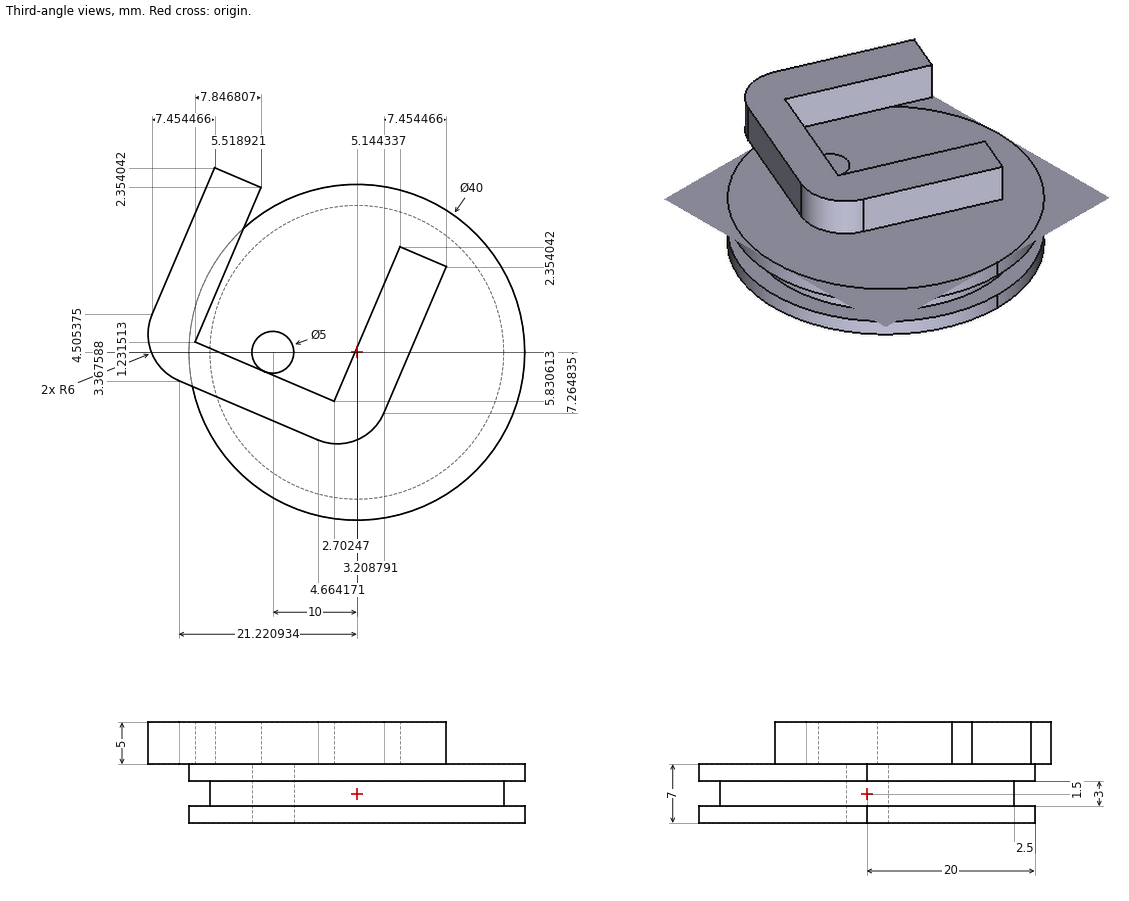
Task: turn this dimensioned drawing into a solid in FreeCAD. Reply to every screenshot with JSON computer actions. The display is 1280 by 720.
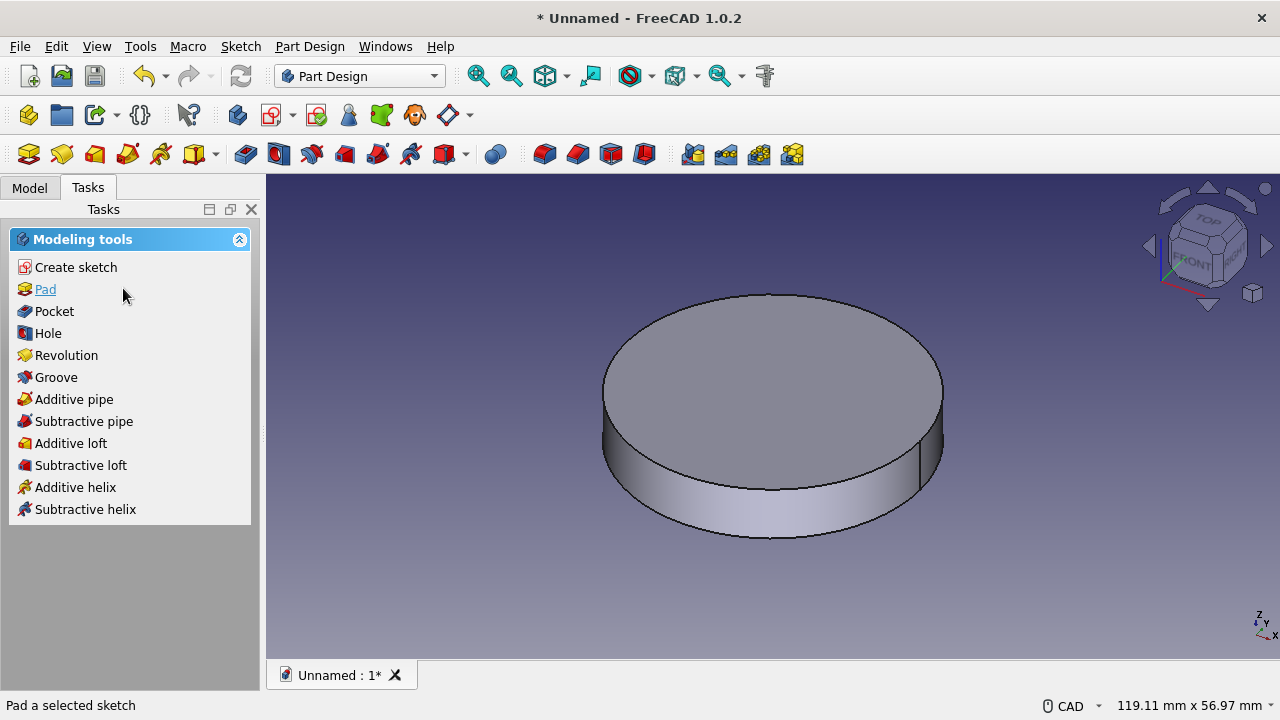
{"action": "left_click", "coordinate": [312, 154]}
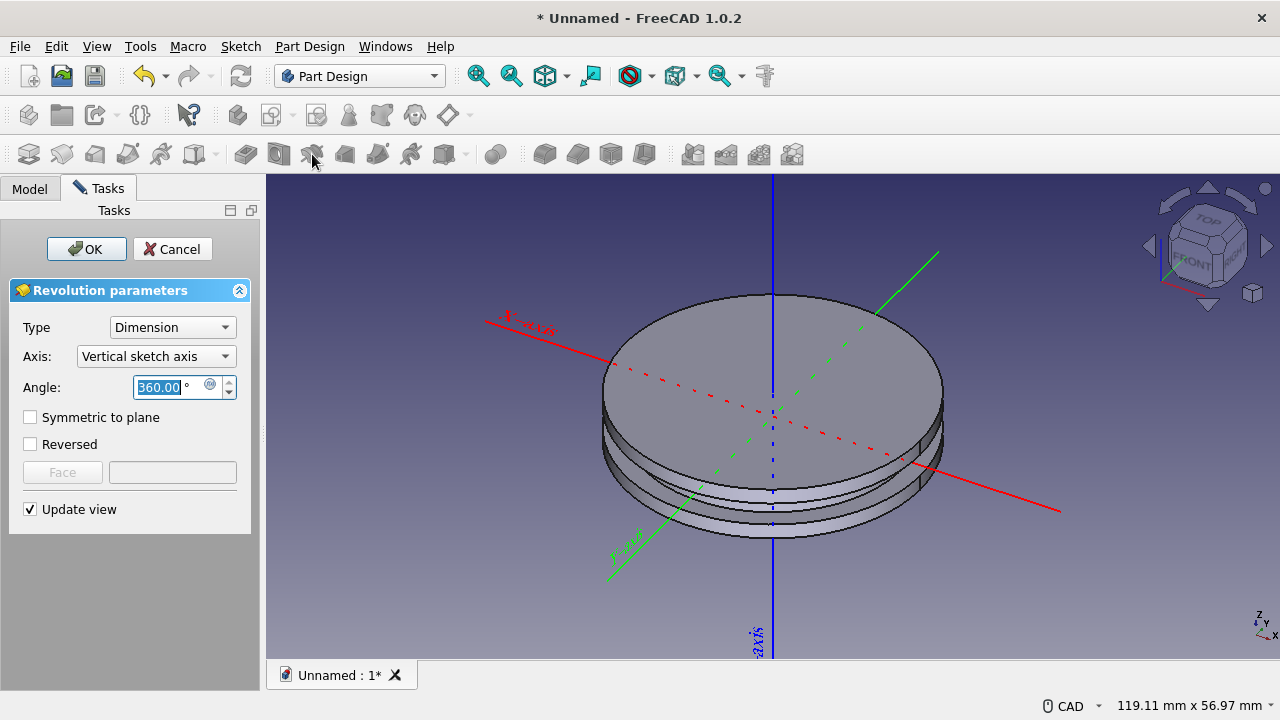
{"action": "left_click", "coordinate": [87, 249]}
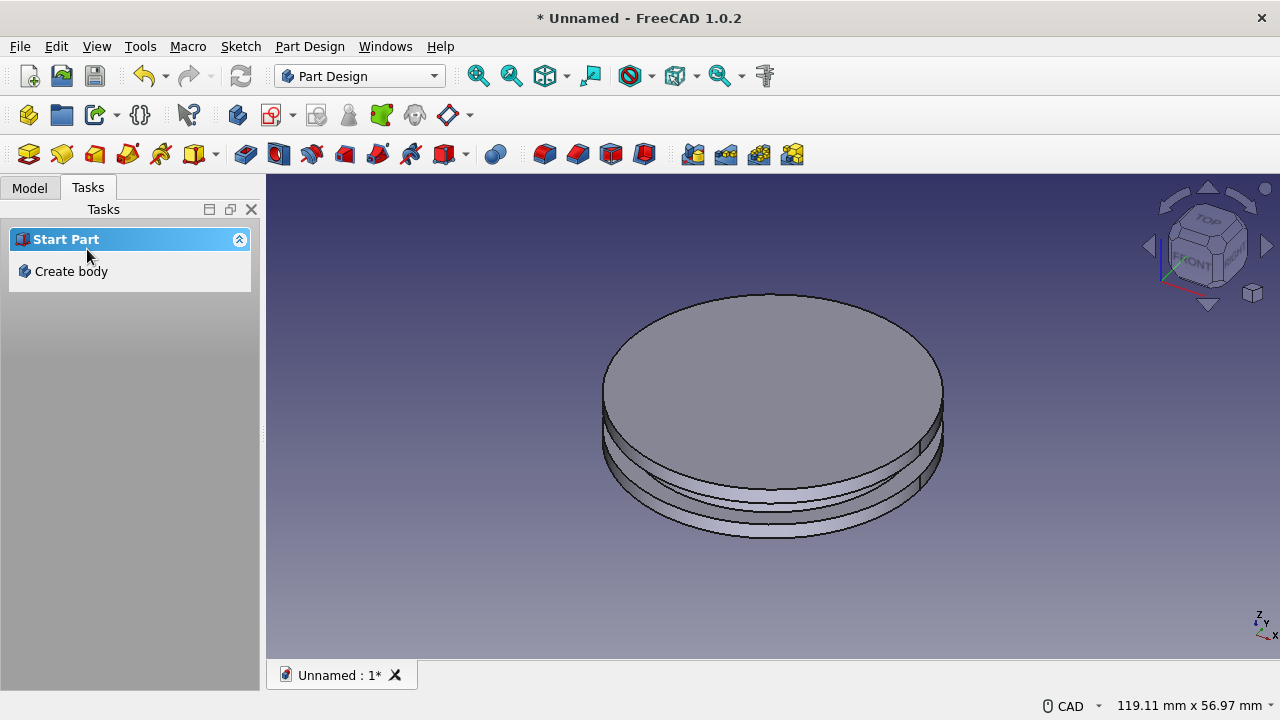
{"action": "left_click", "coordinate": [773, 391]}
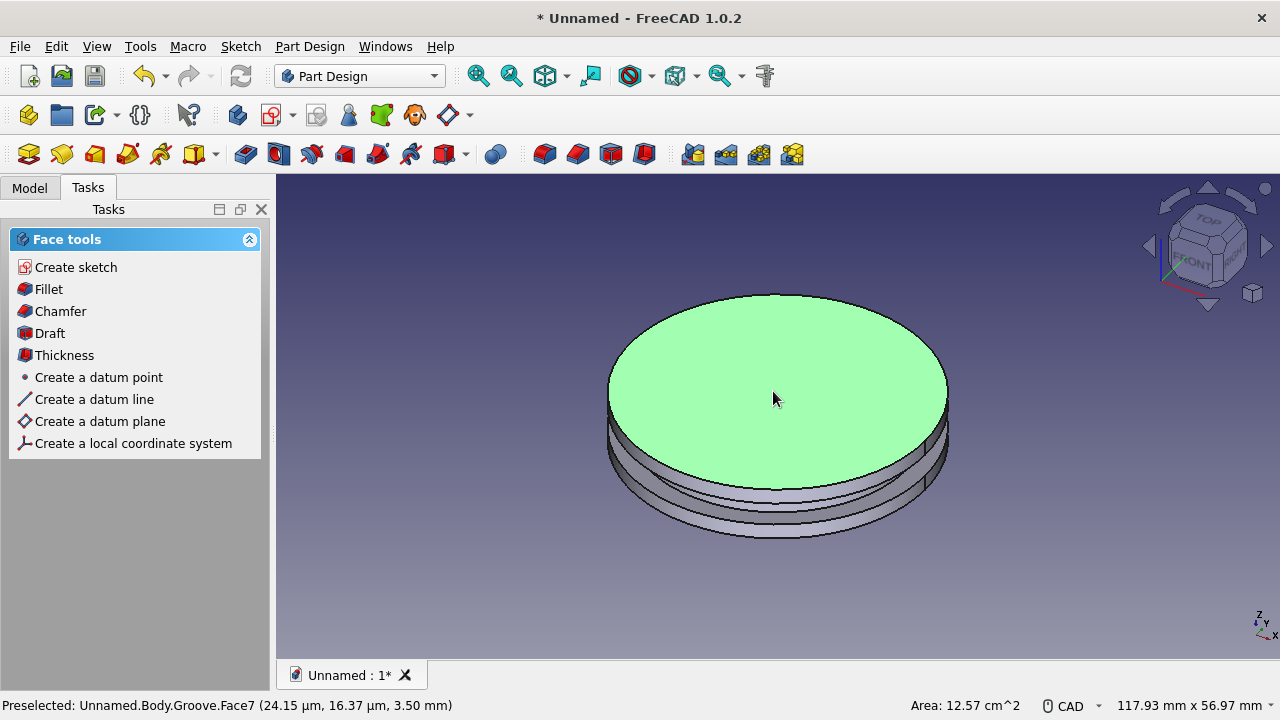
{"action": "left_click", "coordinate": [270, 116]}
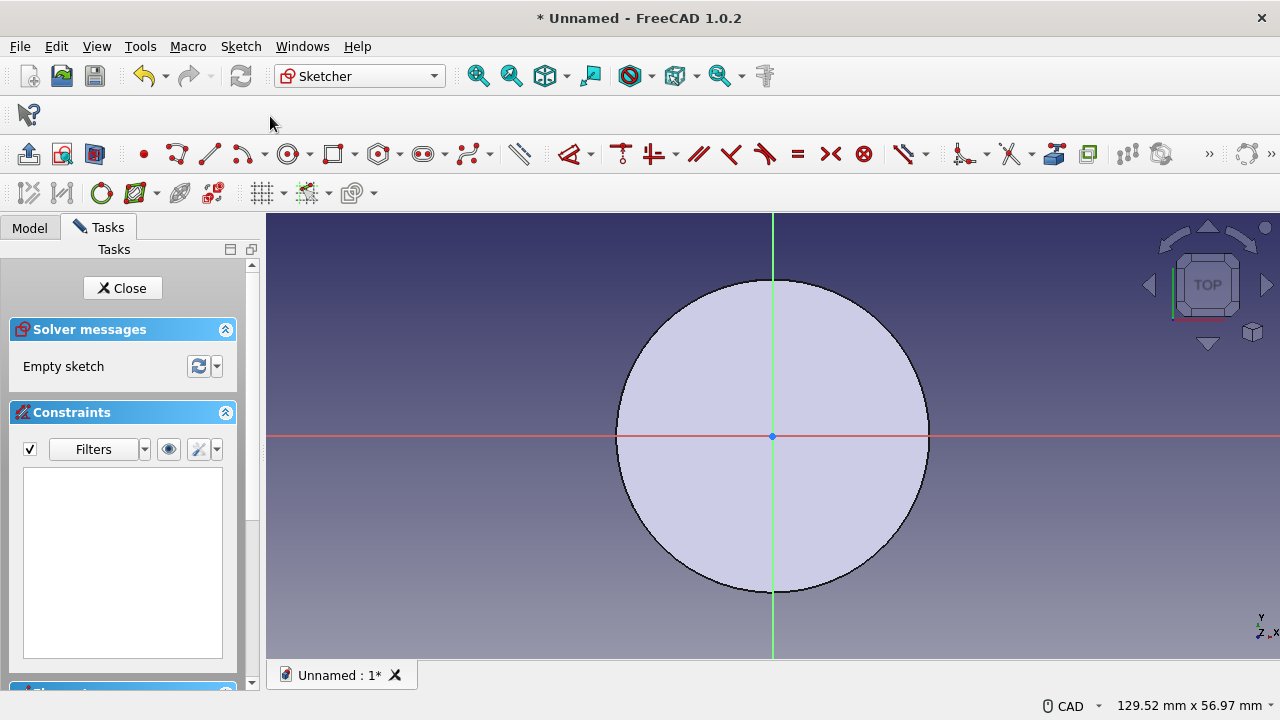
{"action": "scroll", "coordinate": [693, 436], "scroll_direction": "up", "scroll_amount": 10}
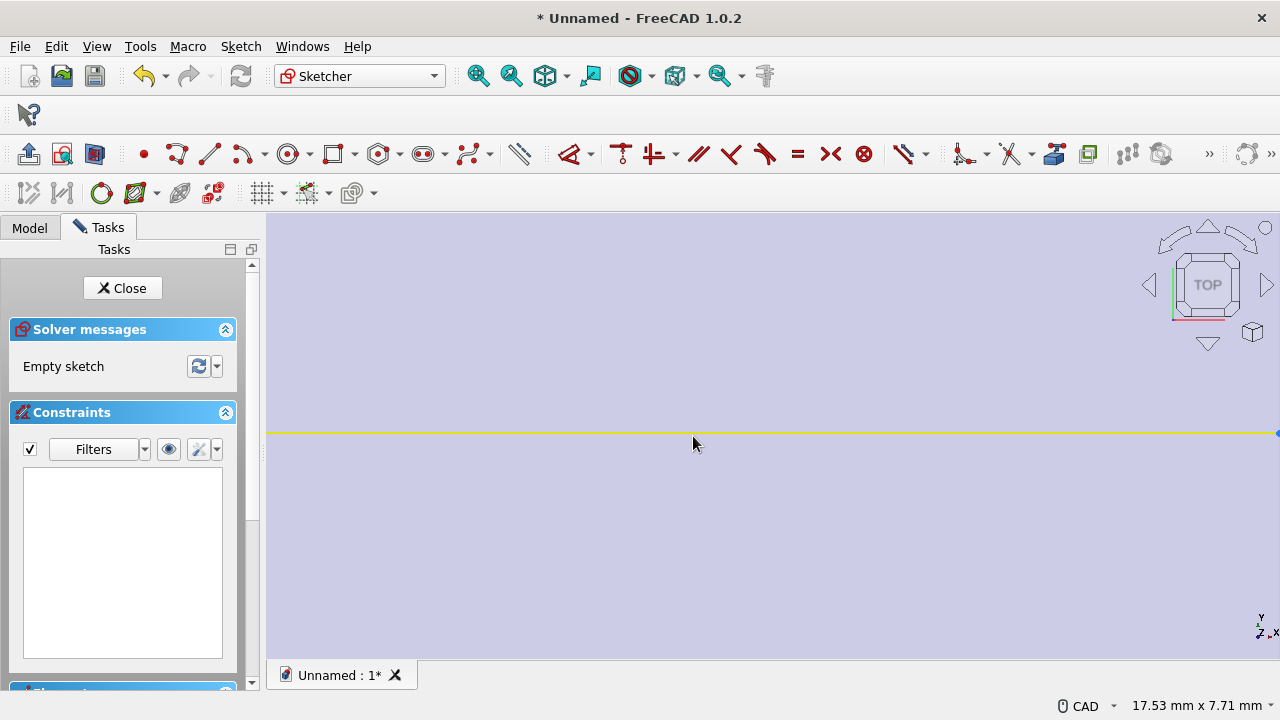
{"action": "left_click", "coordinate": [288, 154]}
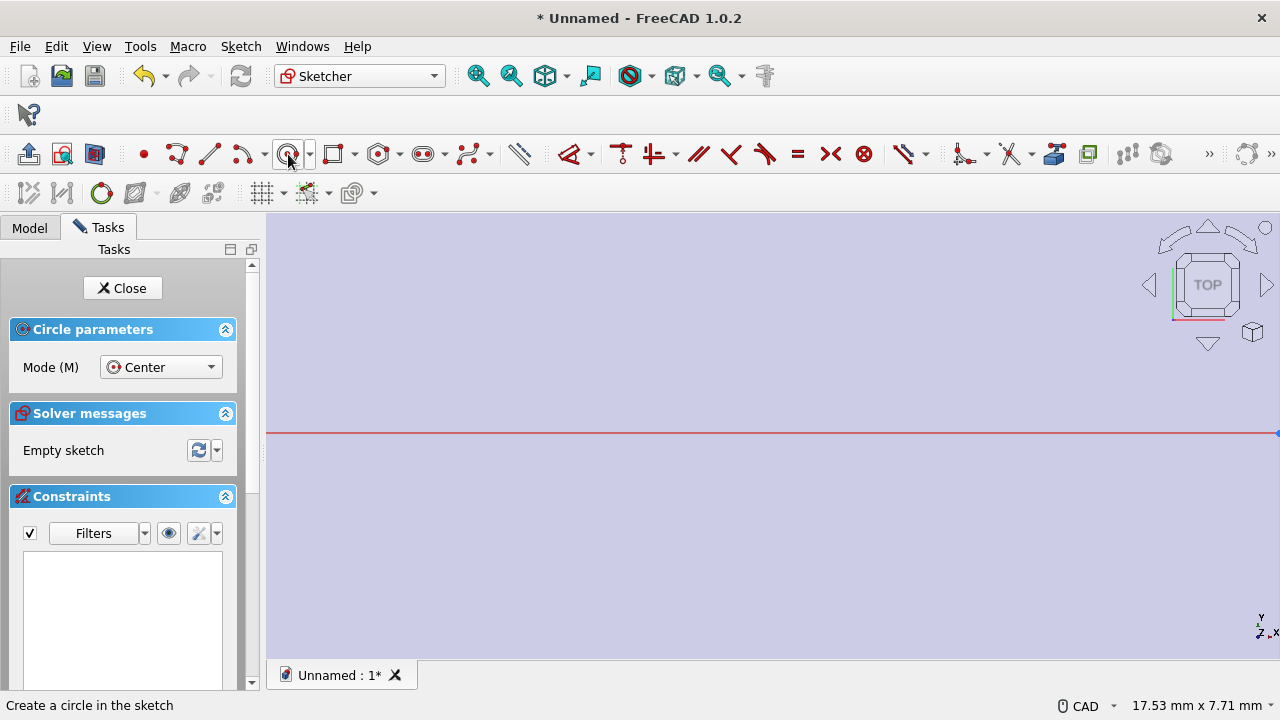
{"action": "left_click", "coordinate": [701, 433]}
{"action": "left_click", "coordinate": [804, 331]}
{"action": "key", "text": "Escape"}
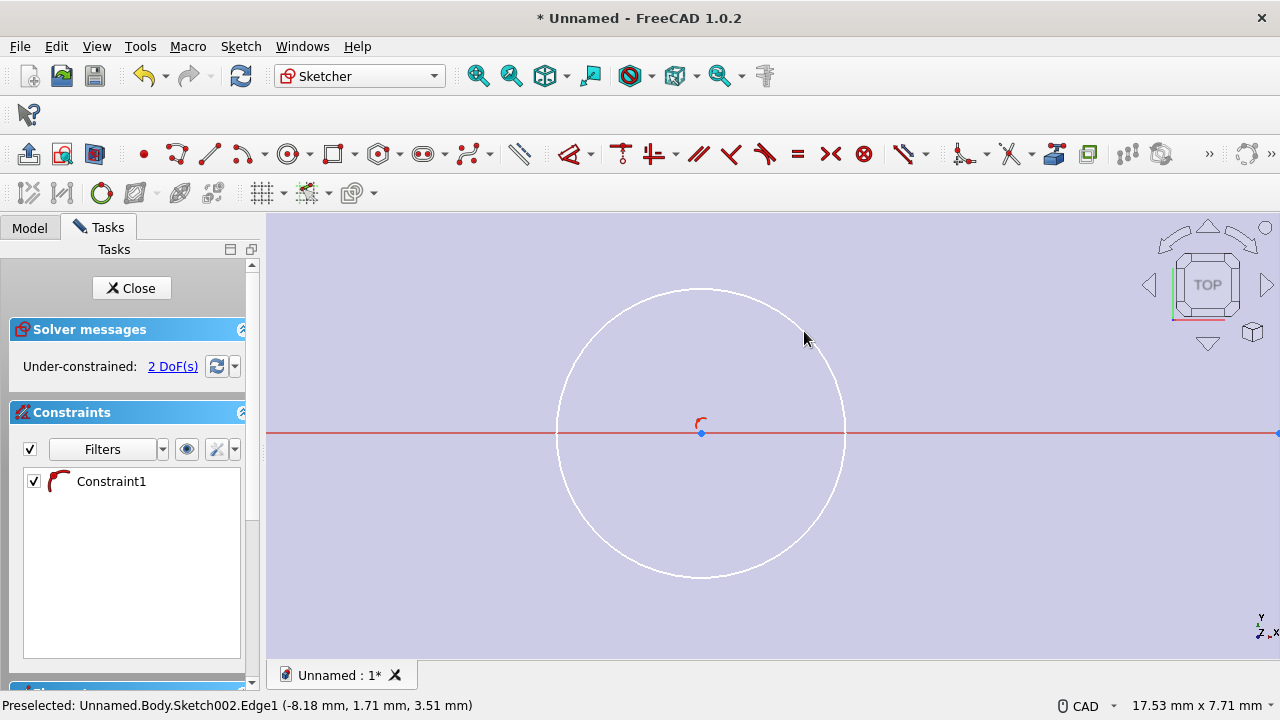
{"action": "left_click", "coordinate": [568, 154]}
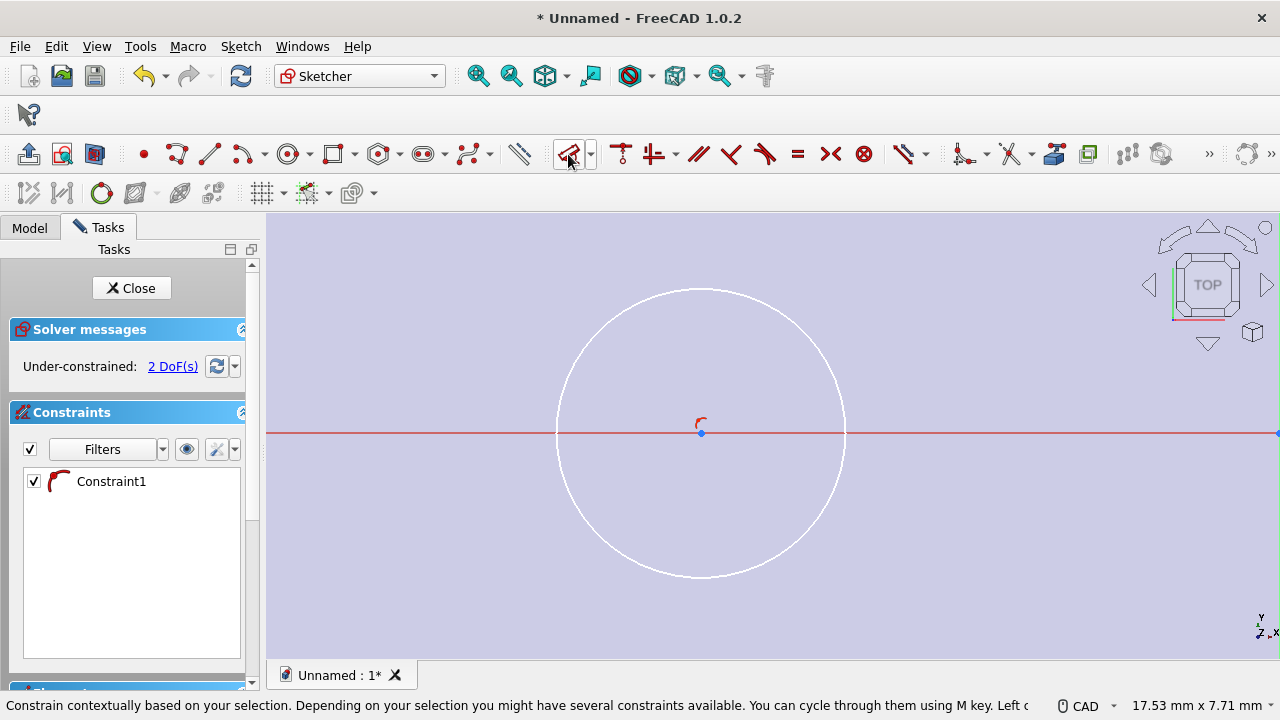
{"action": "left_click", "coordinate": [803, 331]}
{"action": "left_click", "coordinate": [826, 308]}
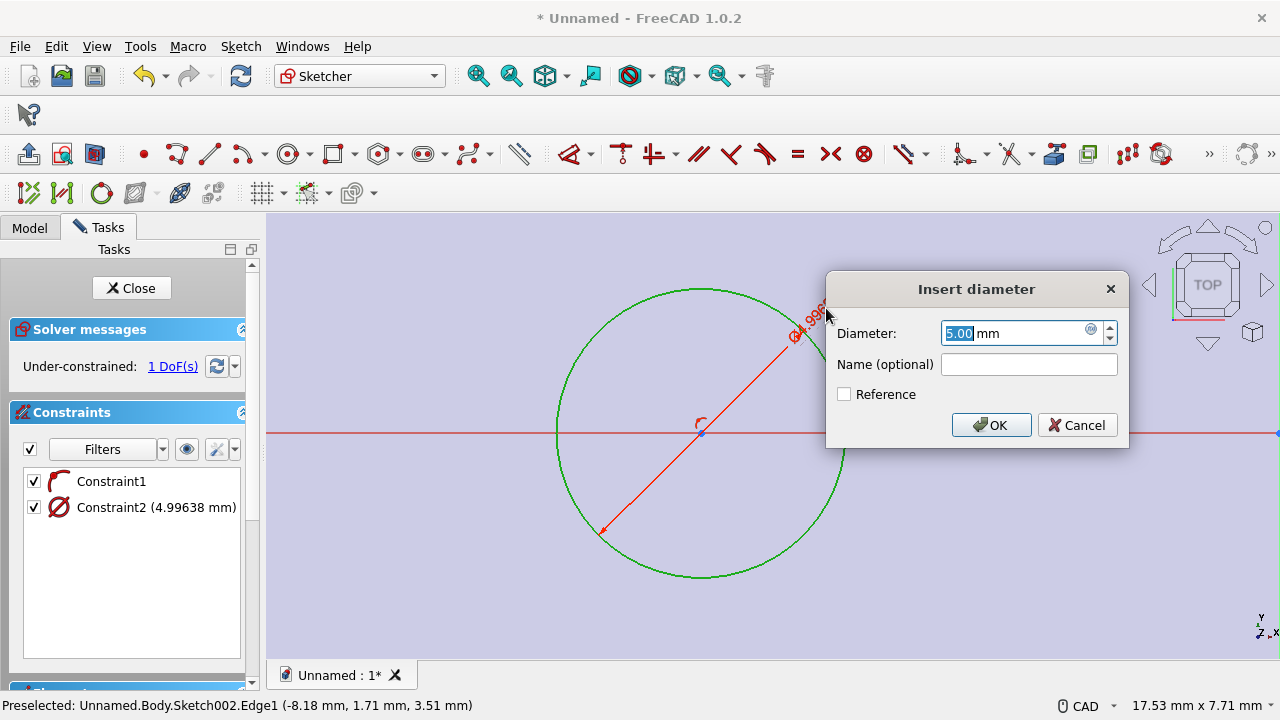
{"action": "type", "text": "5"}
{"action": "key", "text": "Return"}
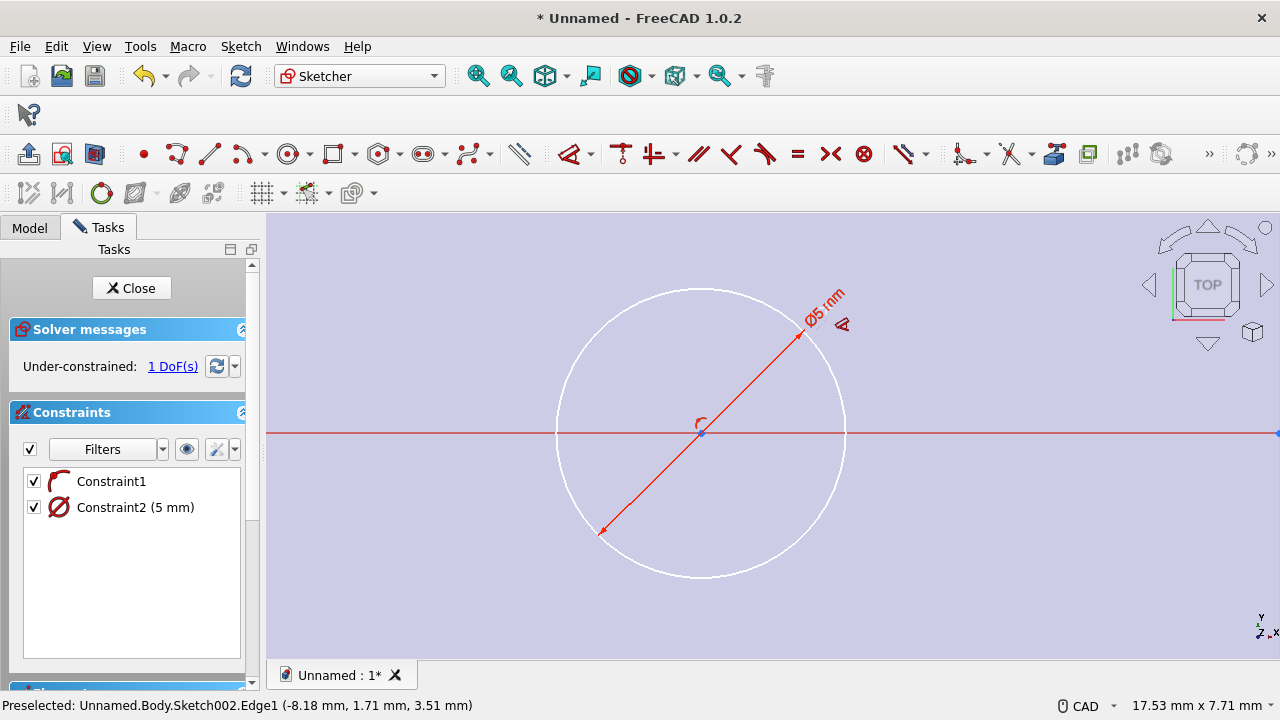
{"action": "left_click", "coordinate": [701, 433]}
{"action": "left_click", "coordinate": [908, 467]}